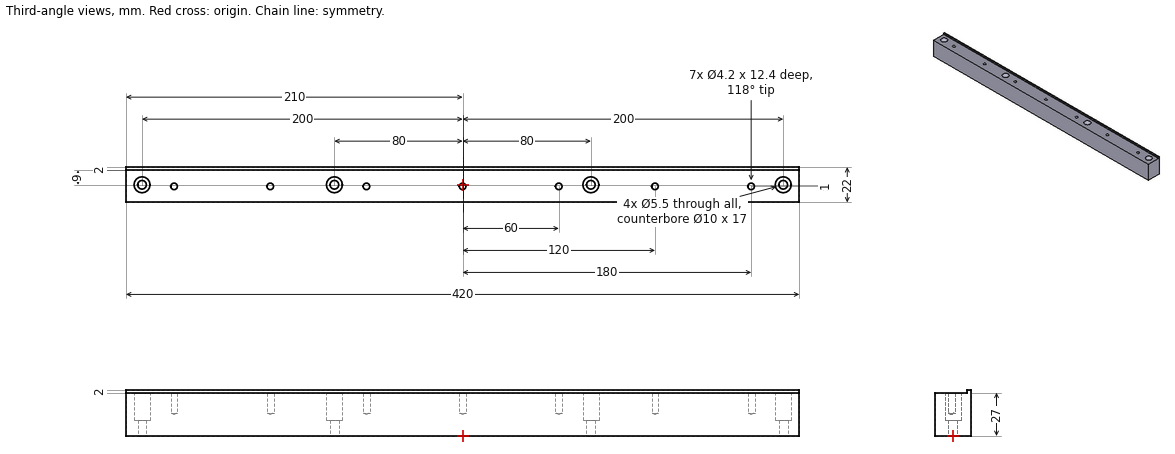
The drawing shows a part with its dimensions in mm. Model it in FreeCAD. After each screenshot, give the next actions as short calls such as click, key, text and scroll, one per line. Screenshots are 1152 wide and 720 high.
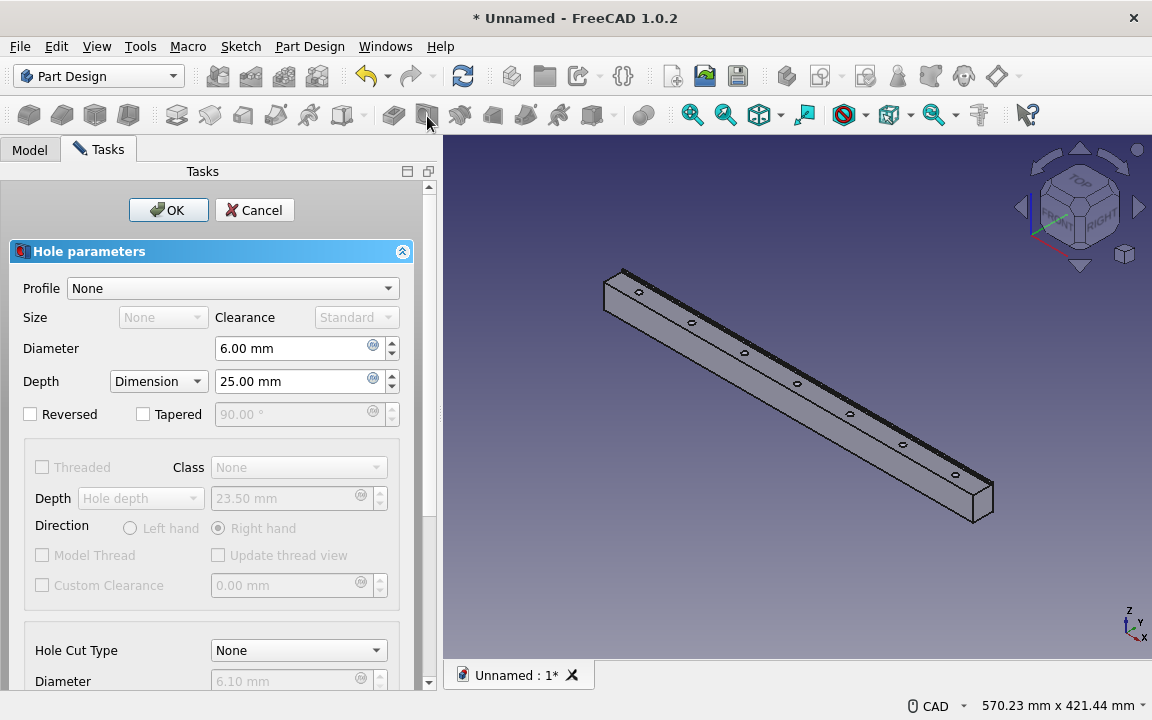
triple_click(300, 348)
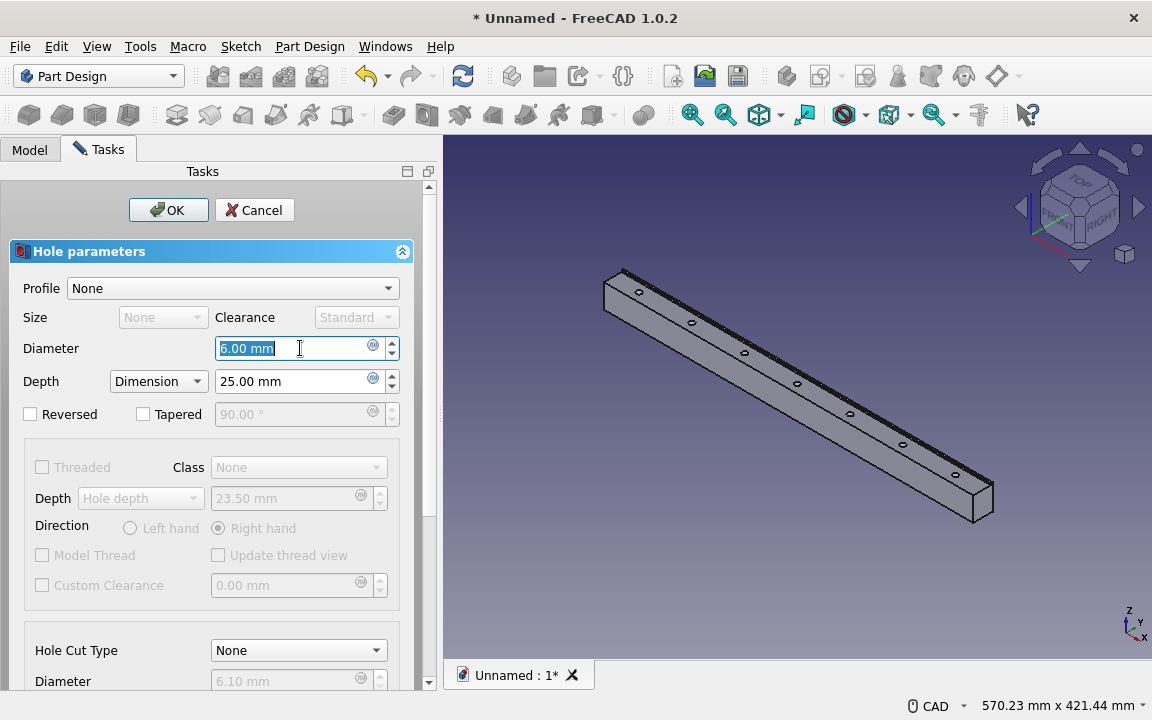
text(4.2)
key(Tab)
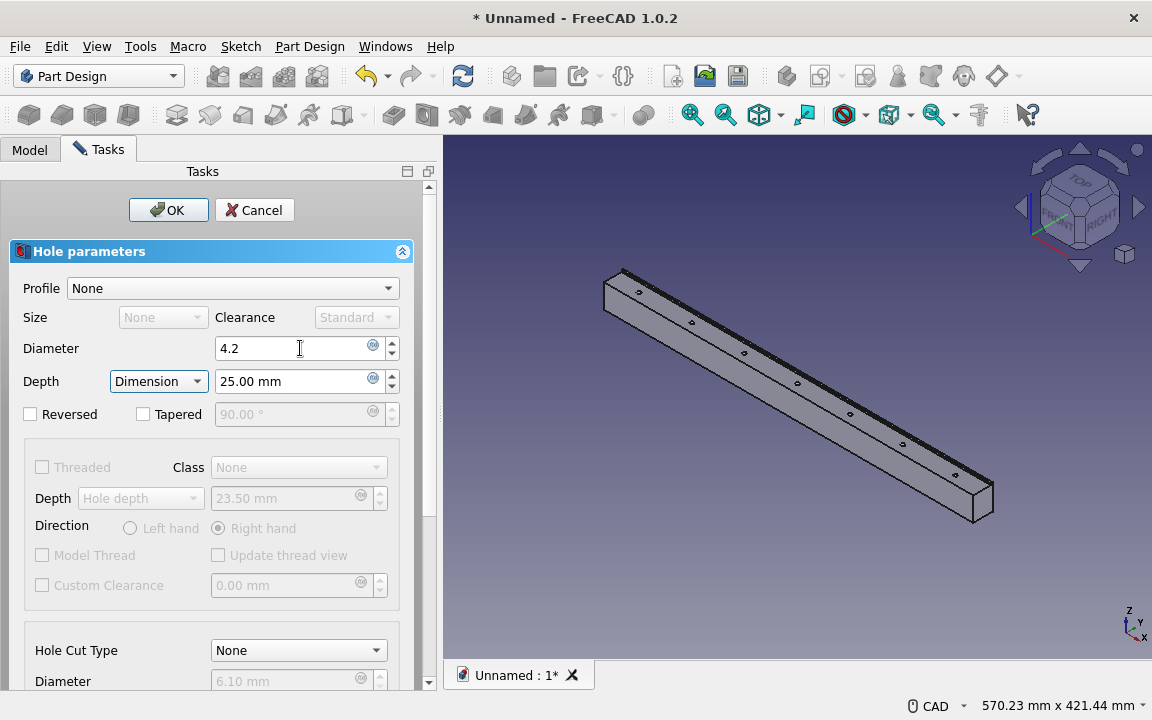
triple_click(300, 382)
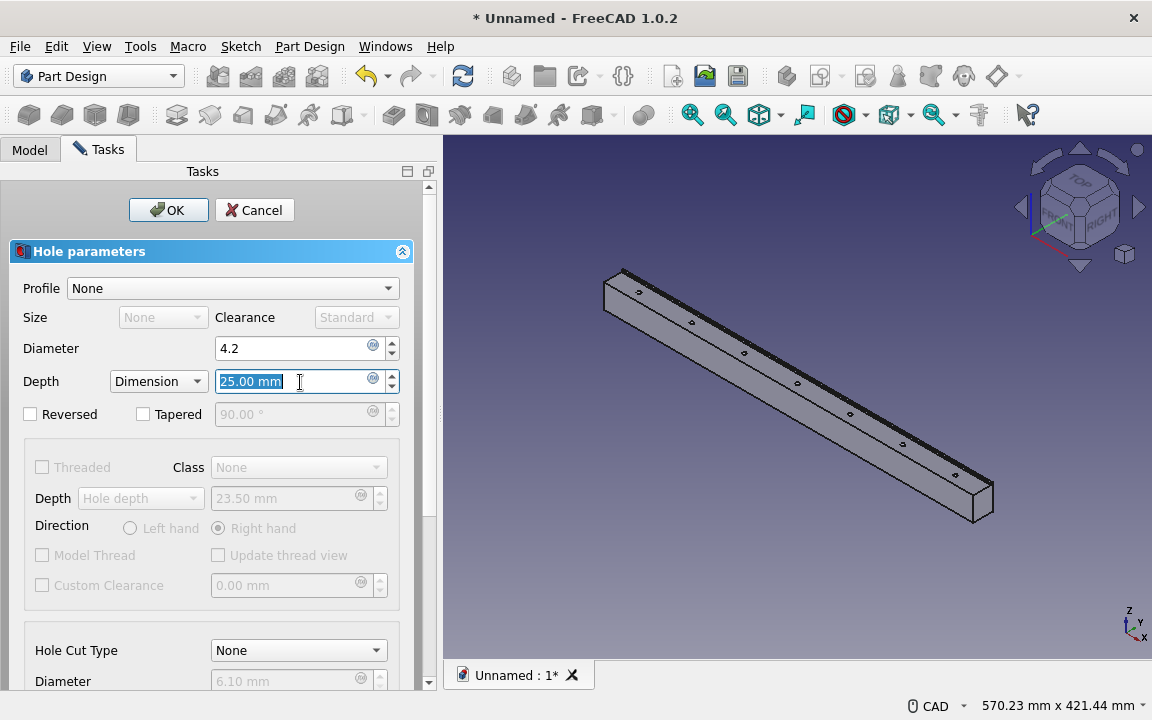
text(12.4)
key(Tab)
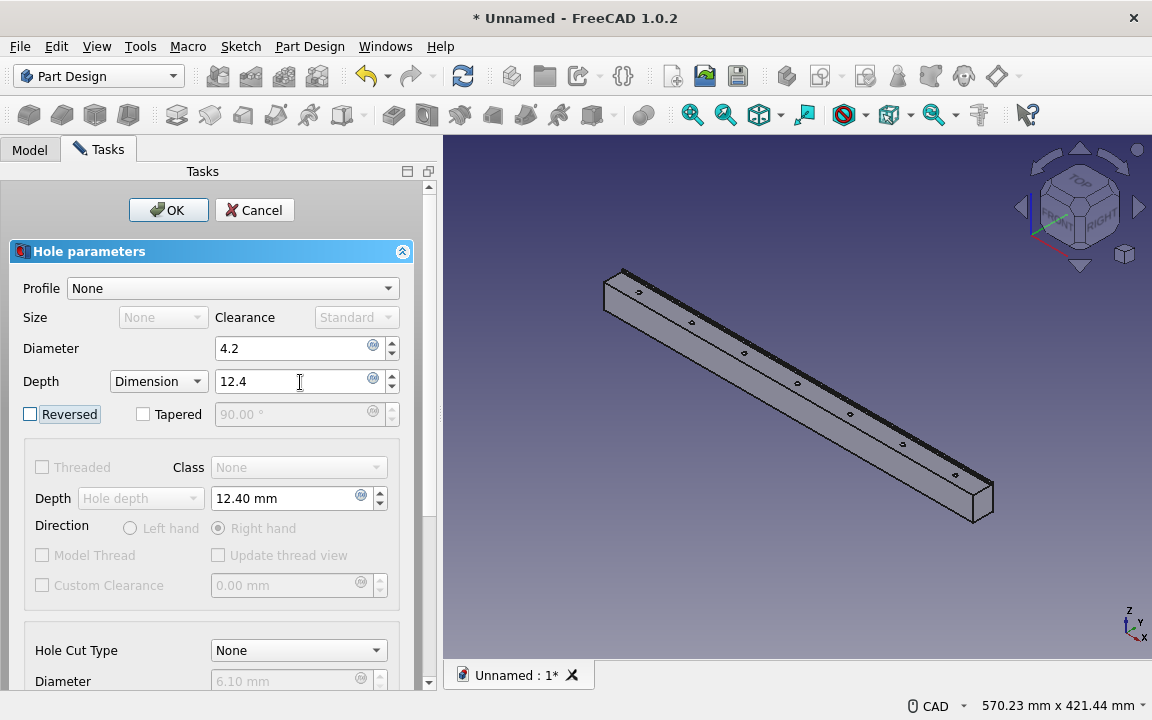
click(169, 210)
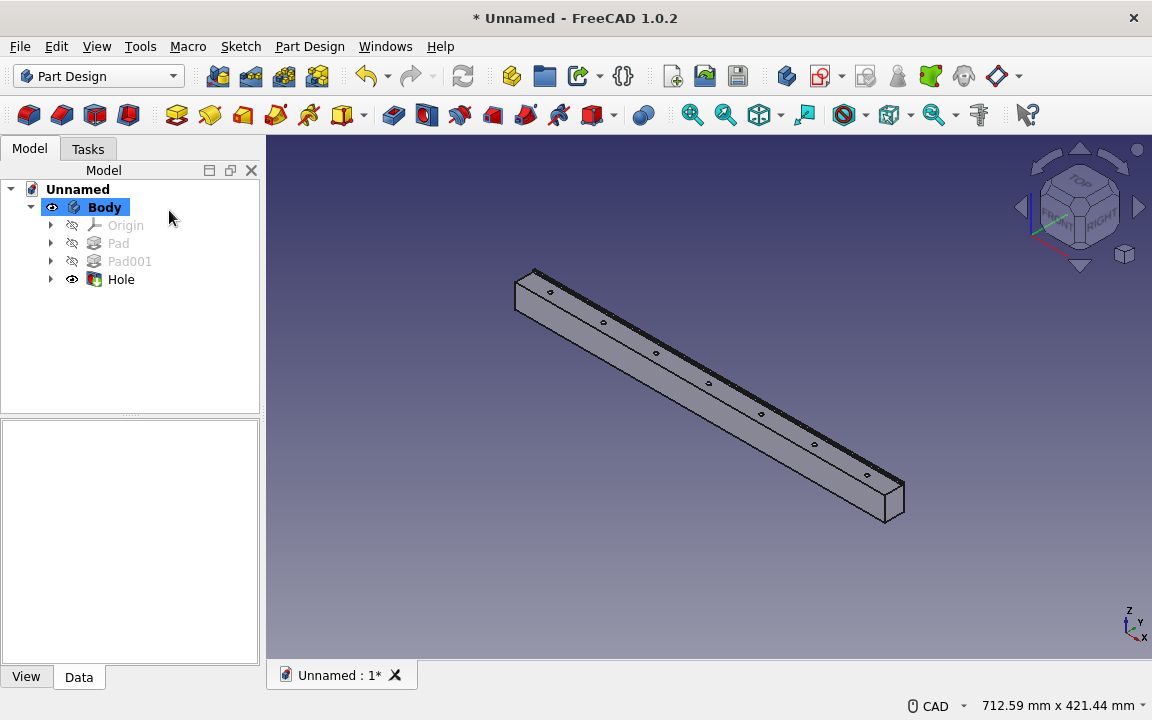
scroll(862, 477, up, 5)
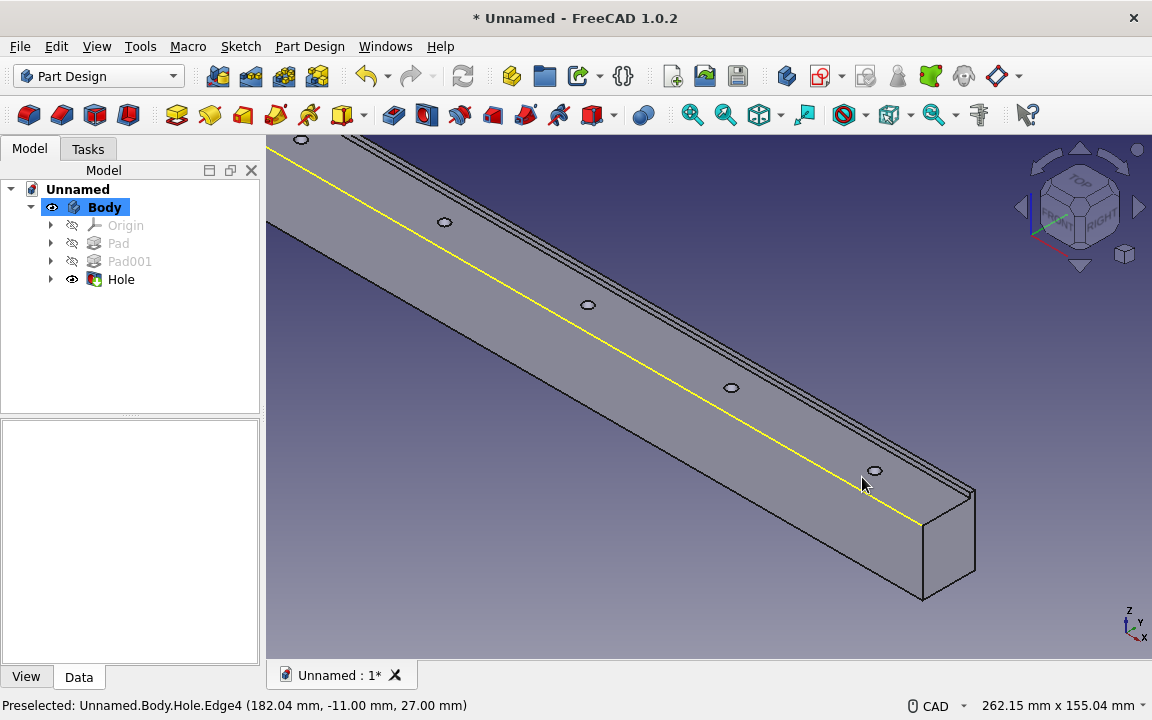
click(861, 478)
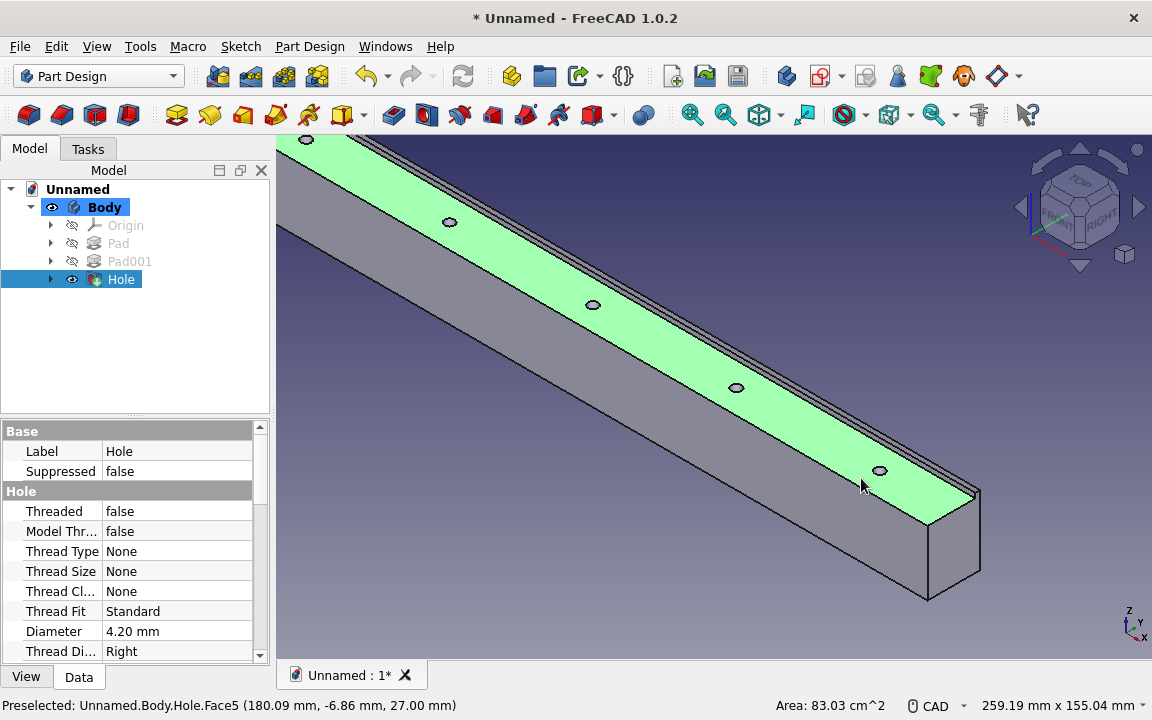
click(820, 76)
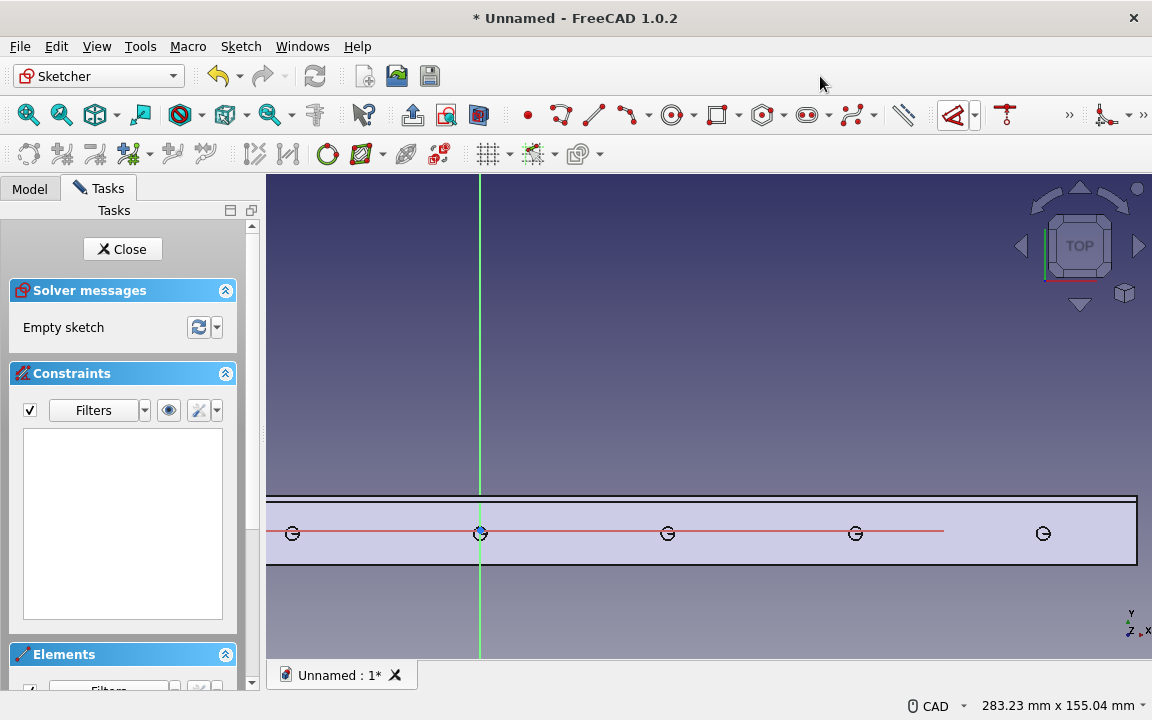
click(479, 116)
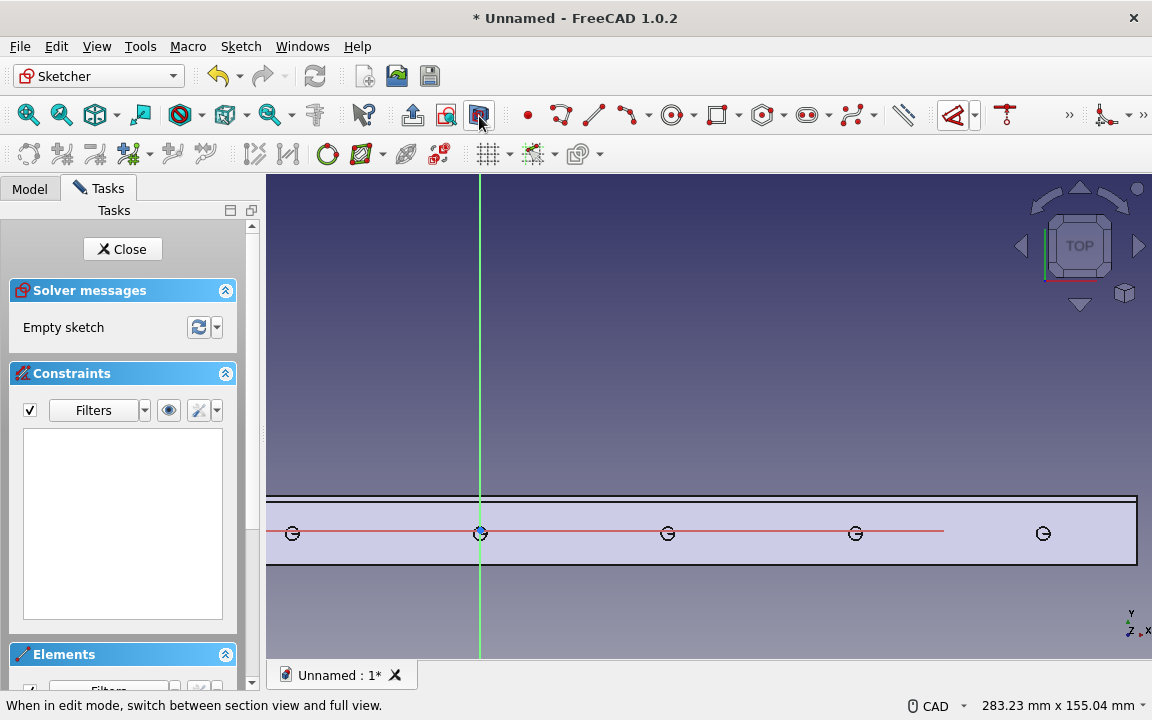
scroll(734, 350, down, 5)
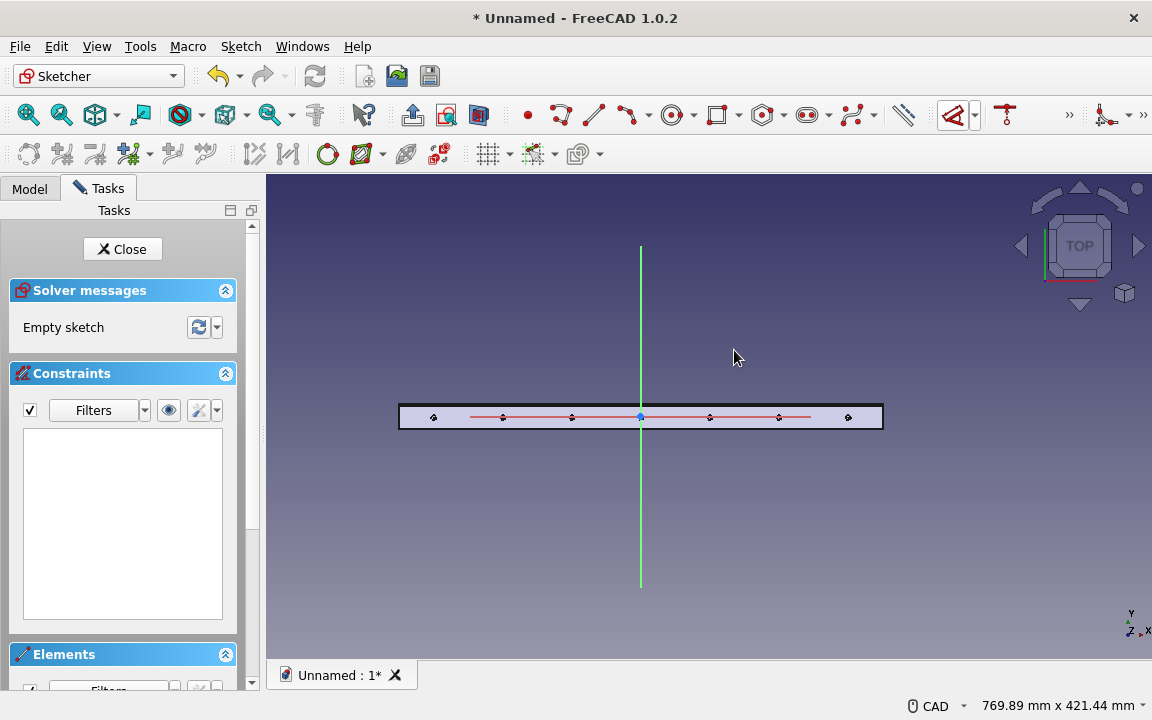
click(672, 116)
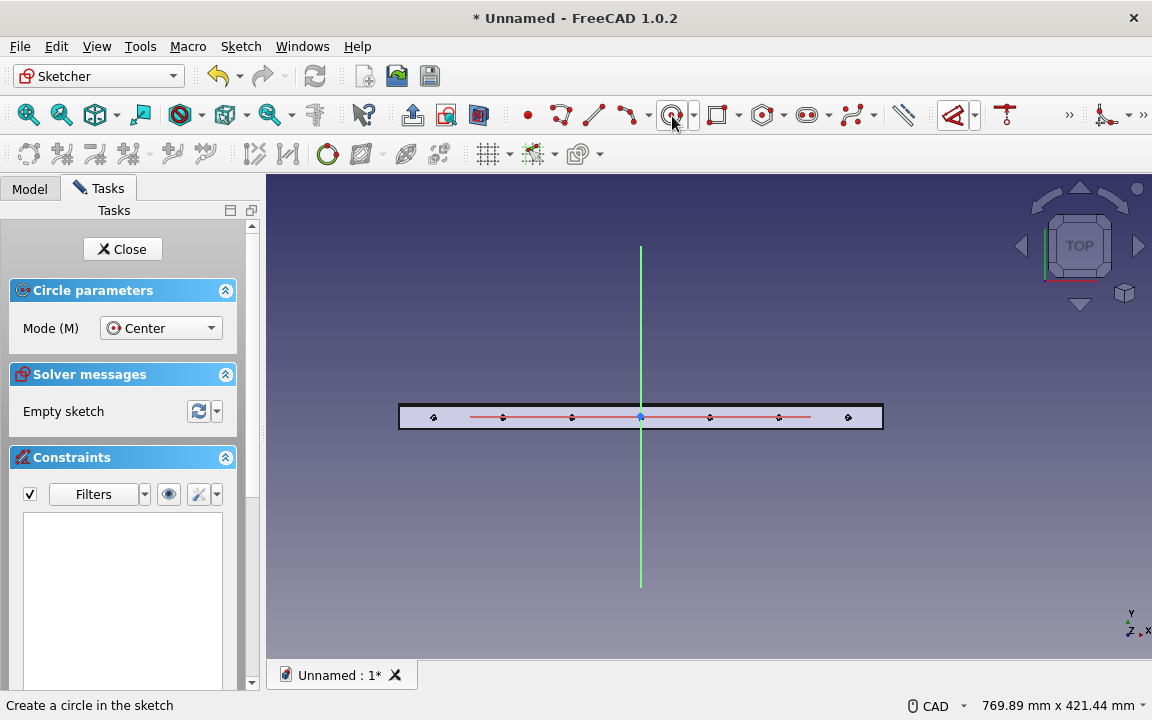
scroll(871, 417, up, 10)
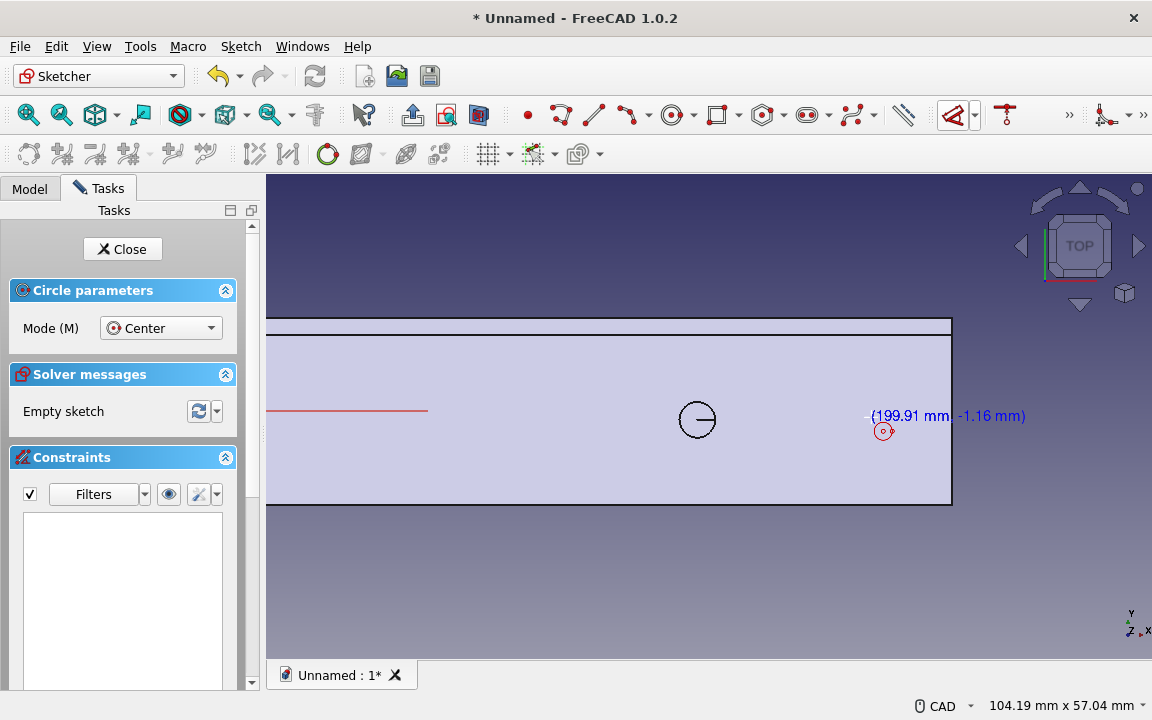
scroll(871, 417, down, 10)